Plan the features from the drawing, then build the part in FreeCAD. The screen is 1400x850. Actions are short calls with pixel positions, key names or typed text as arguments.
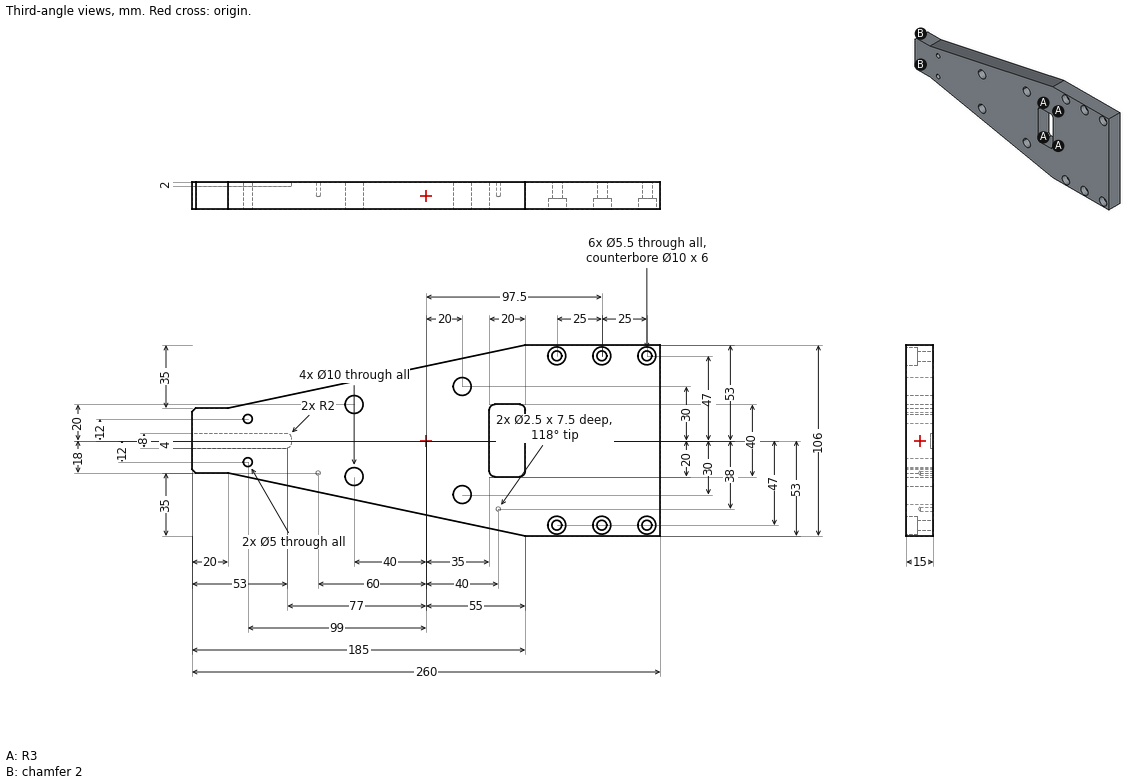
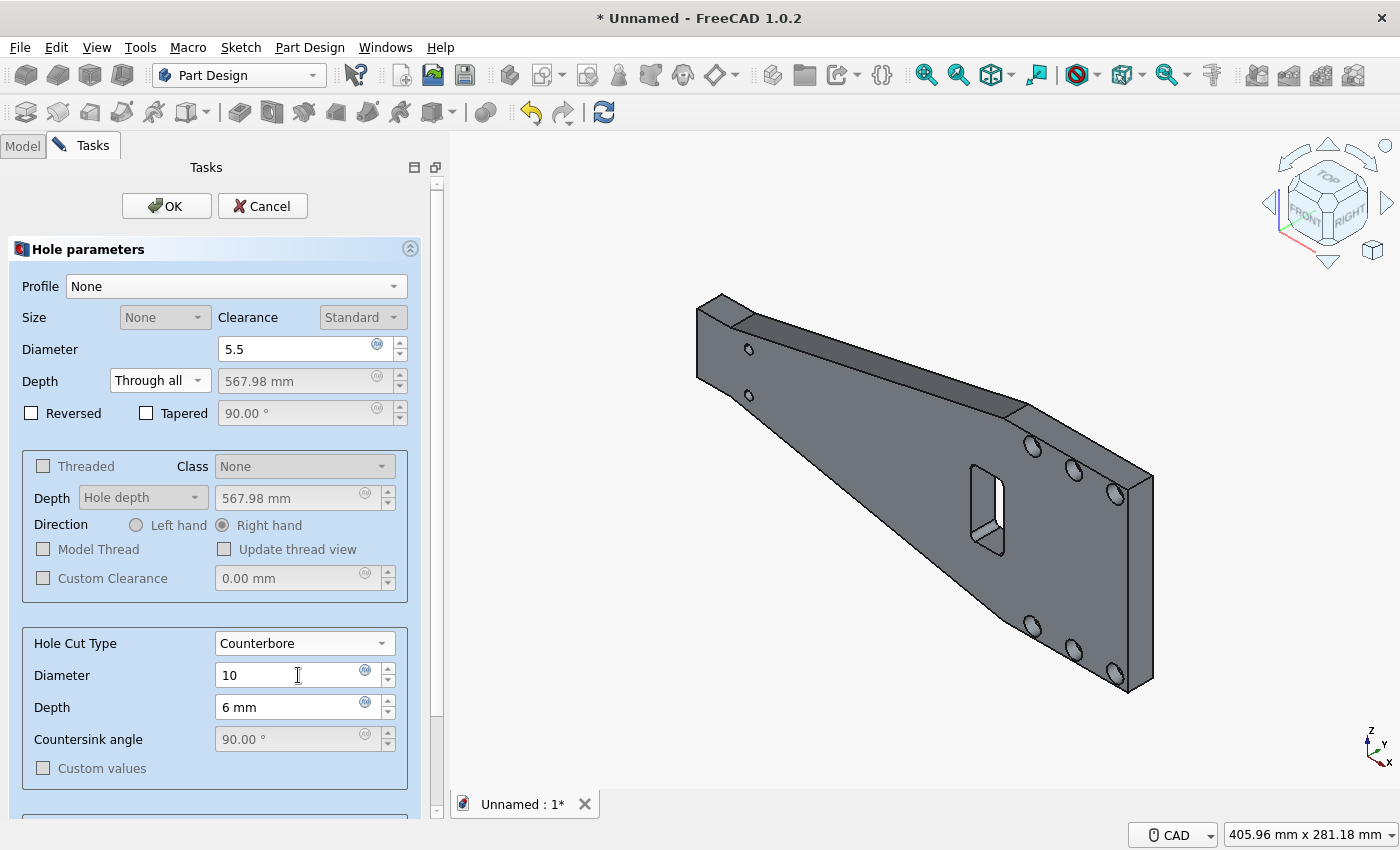
click(167, 206)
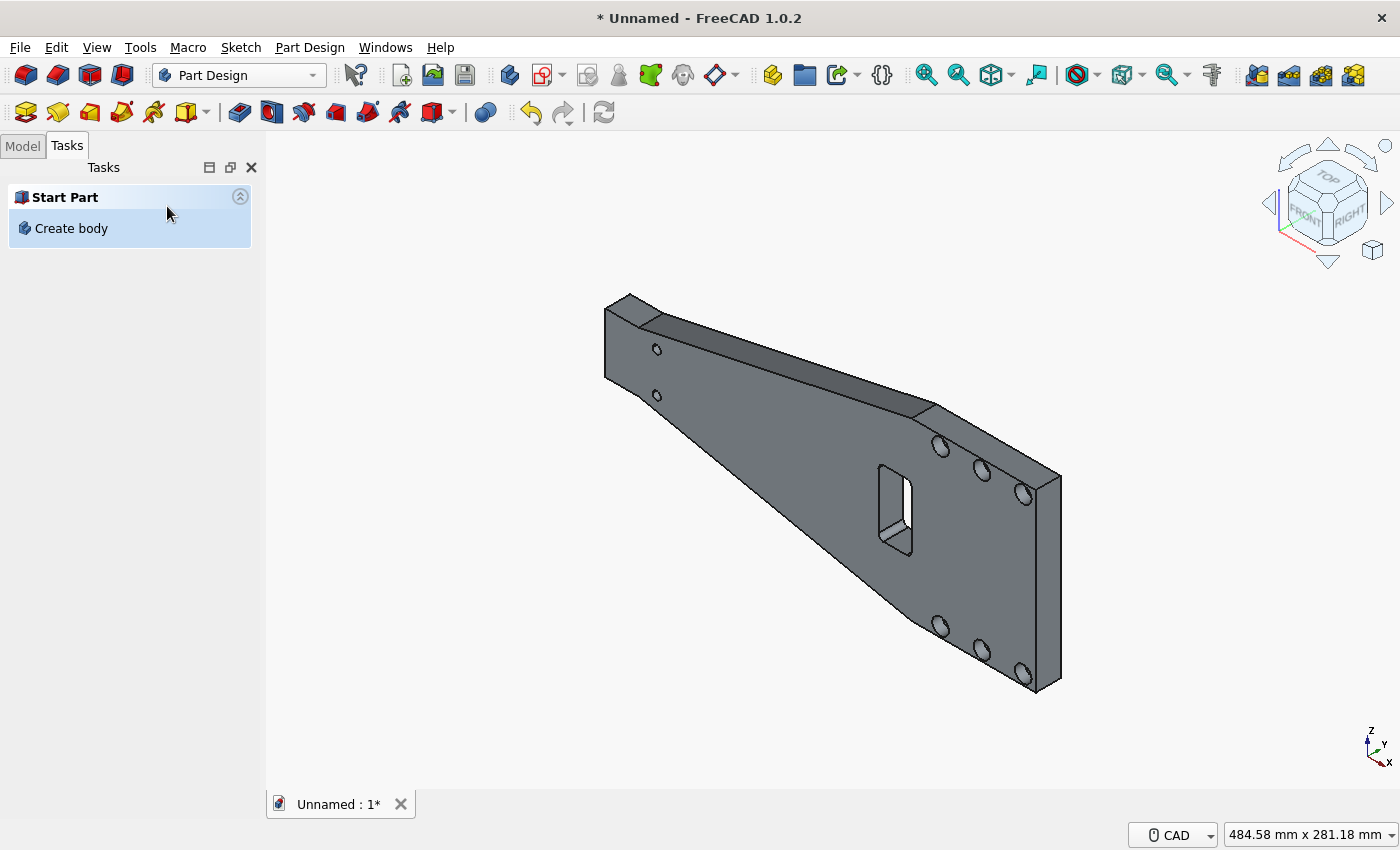
key(2)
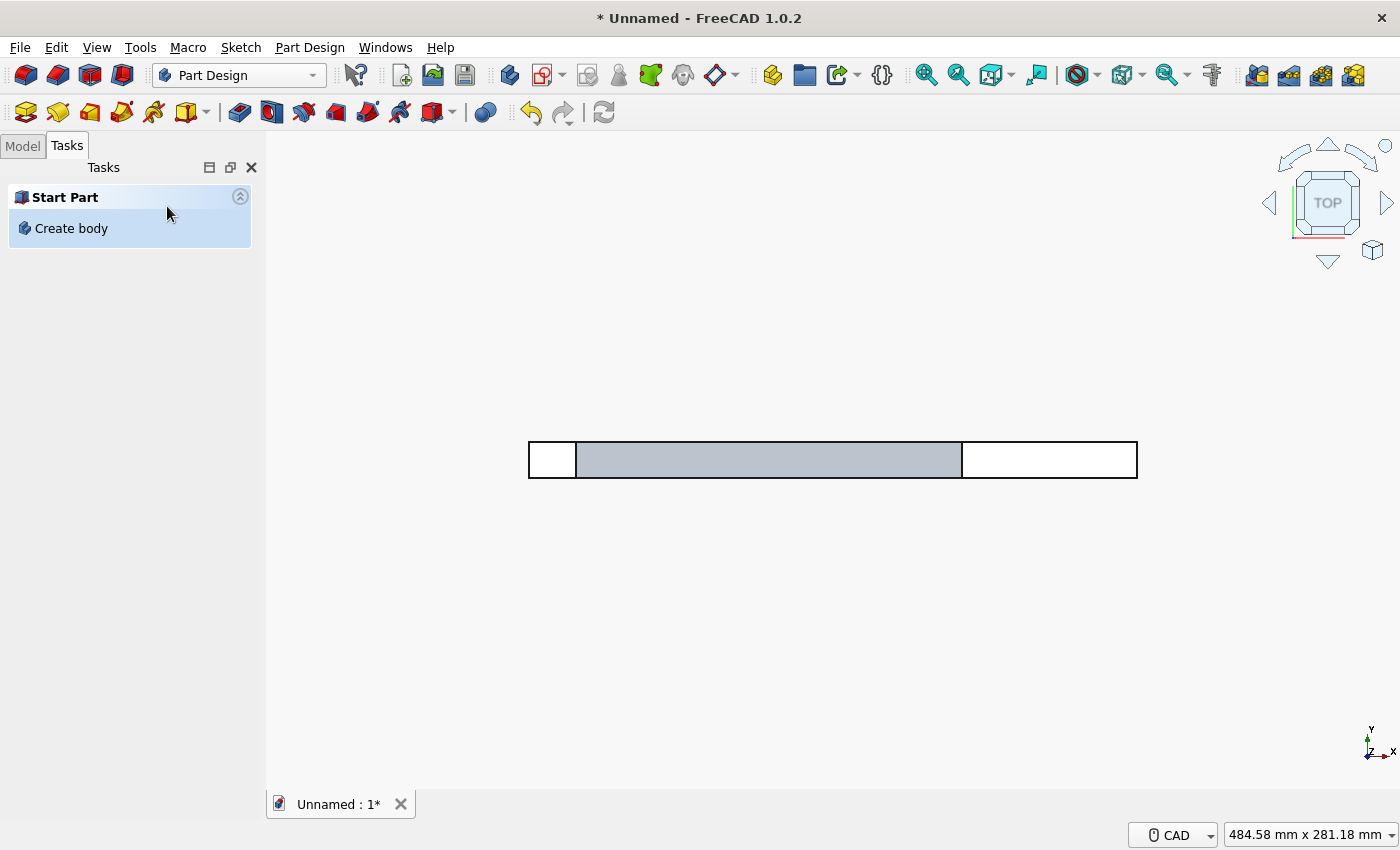
click(529, 459)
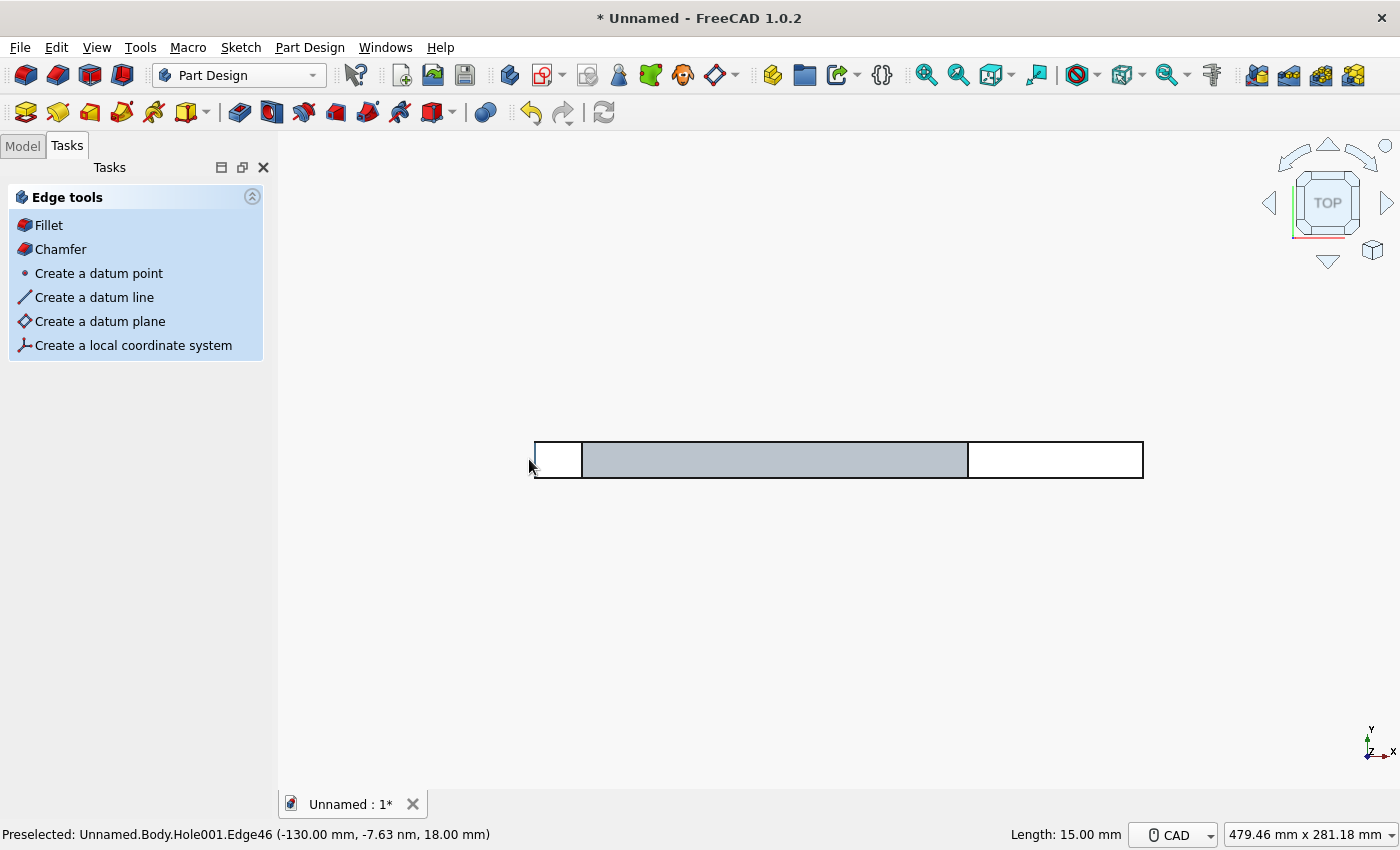
key(0)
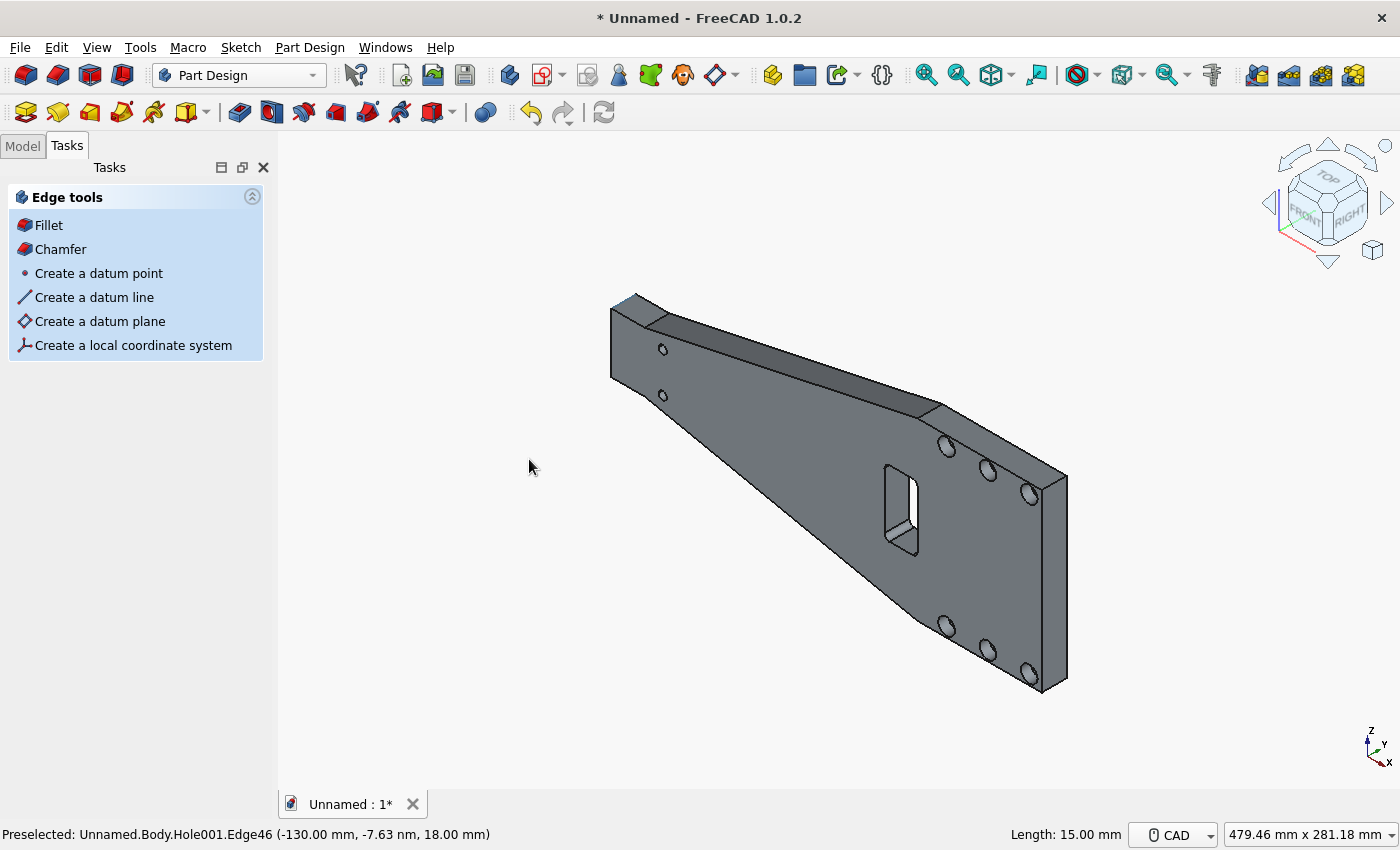
key(1)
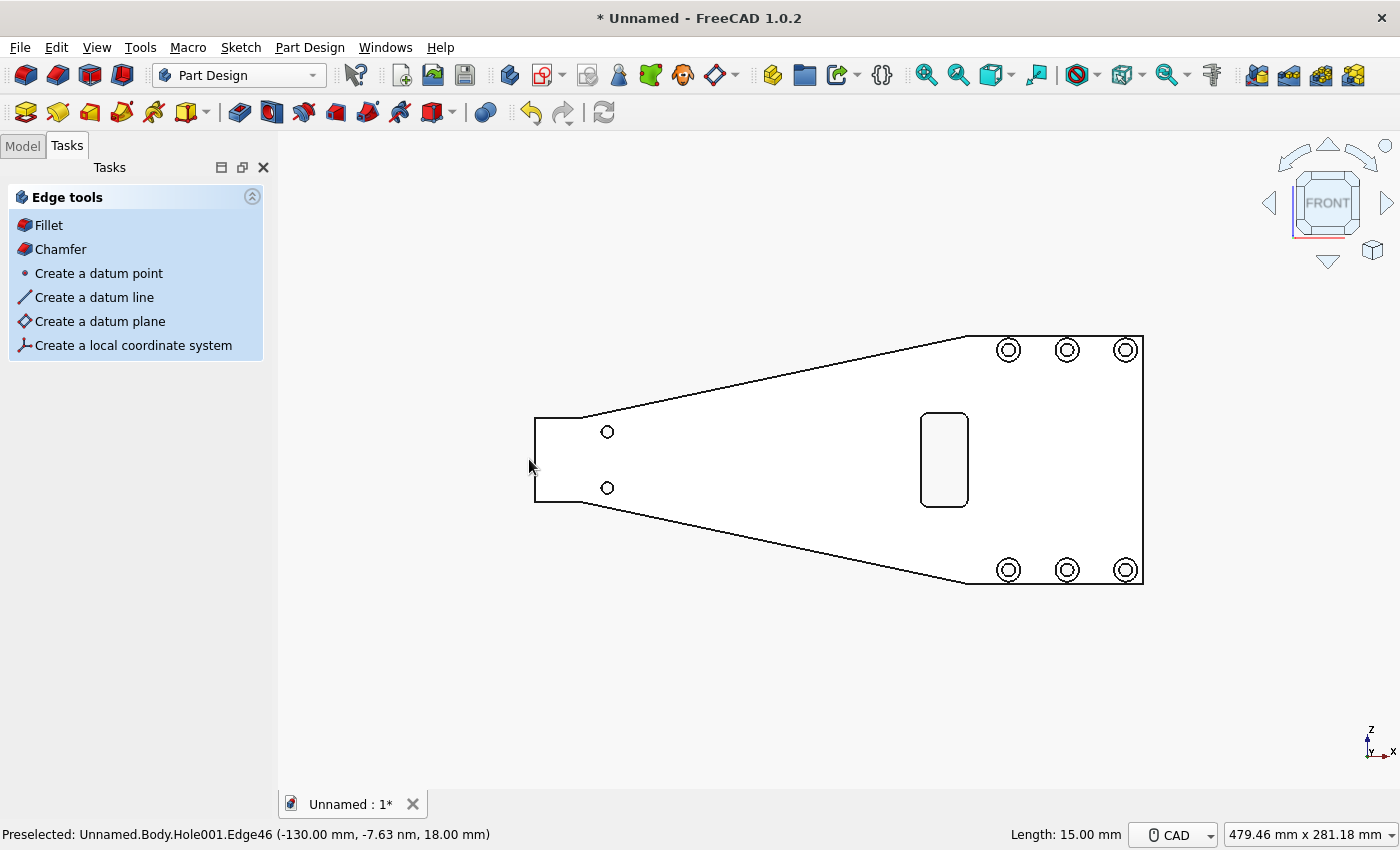
key(3)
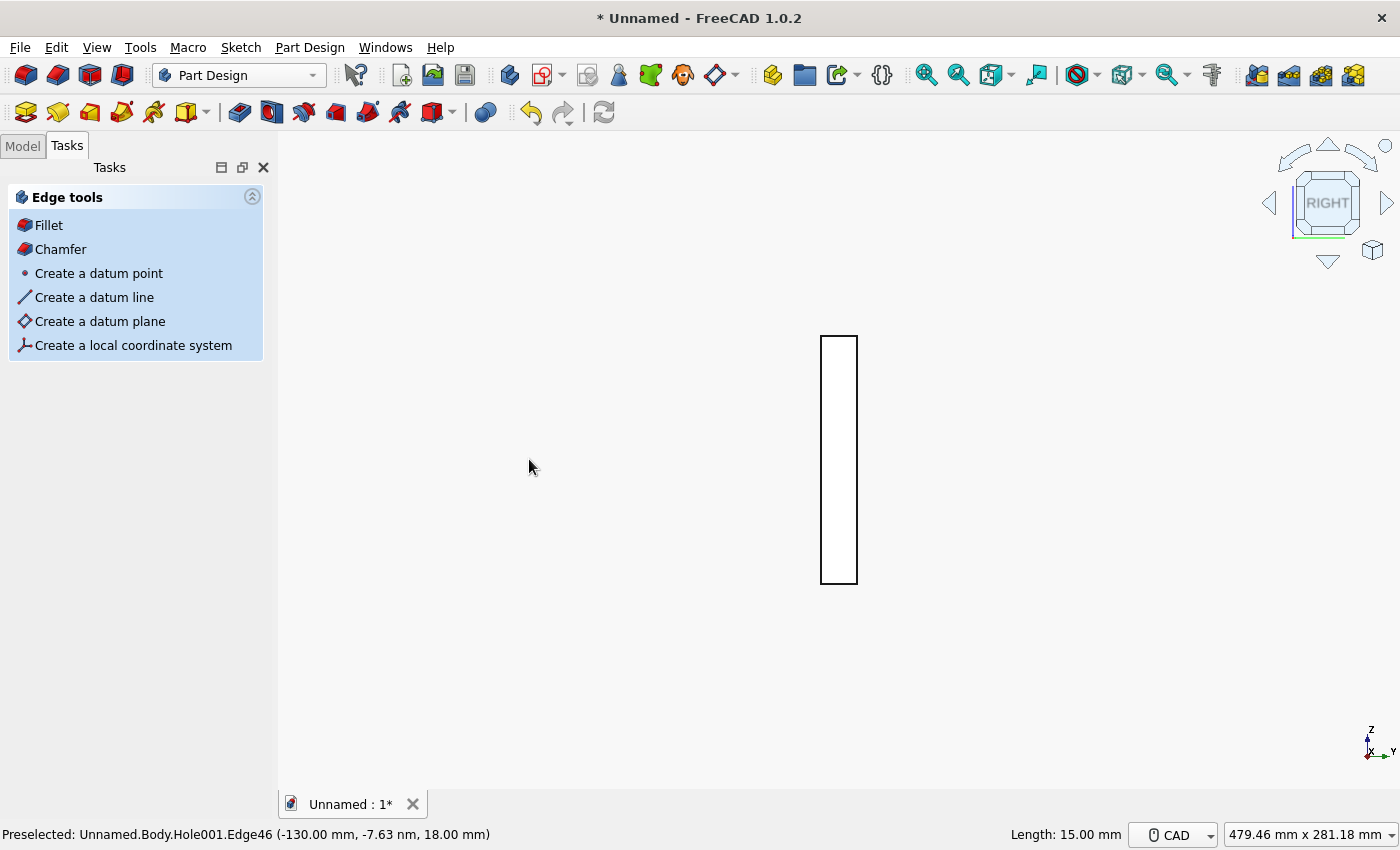
click(928, 76)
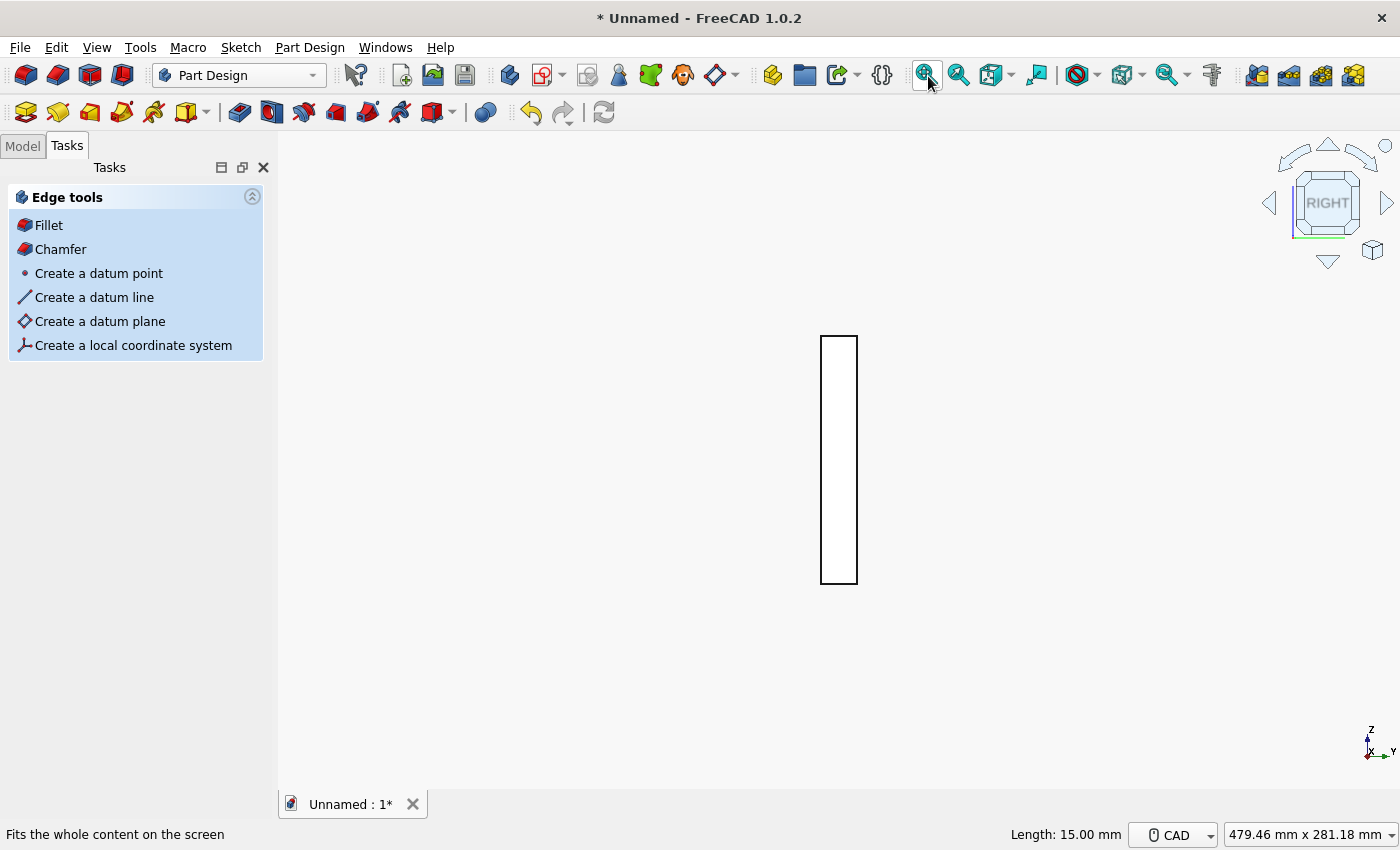
key(5)